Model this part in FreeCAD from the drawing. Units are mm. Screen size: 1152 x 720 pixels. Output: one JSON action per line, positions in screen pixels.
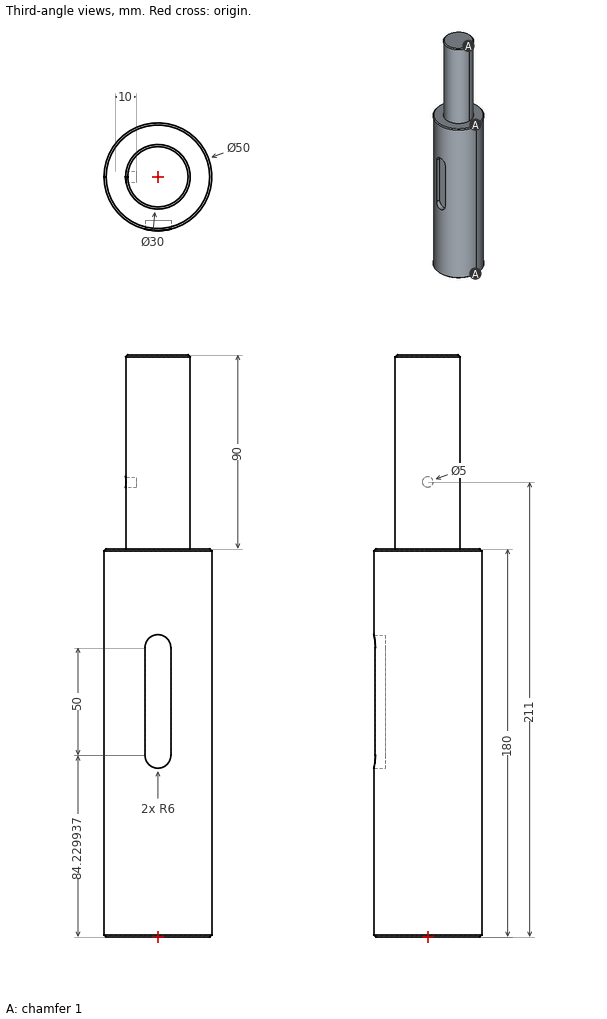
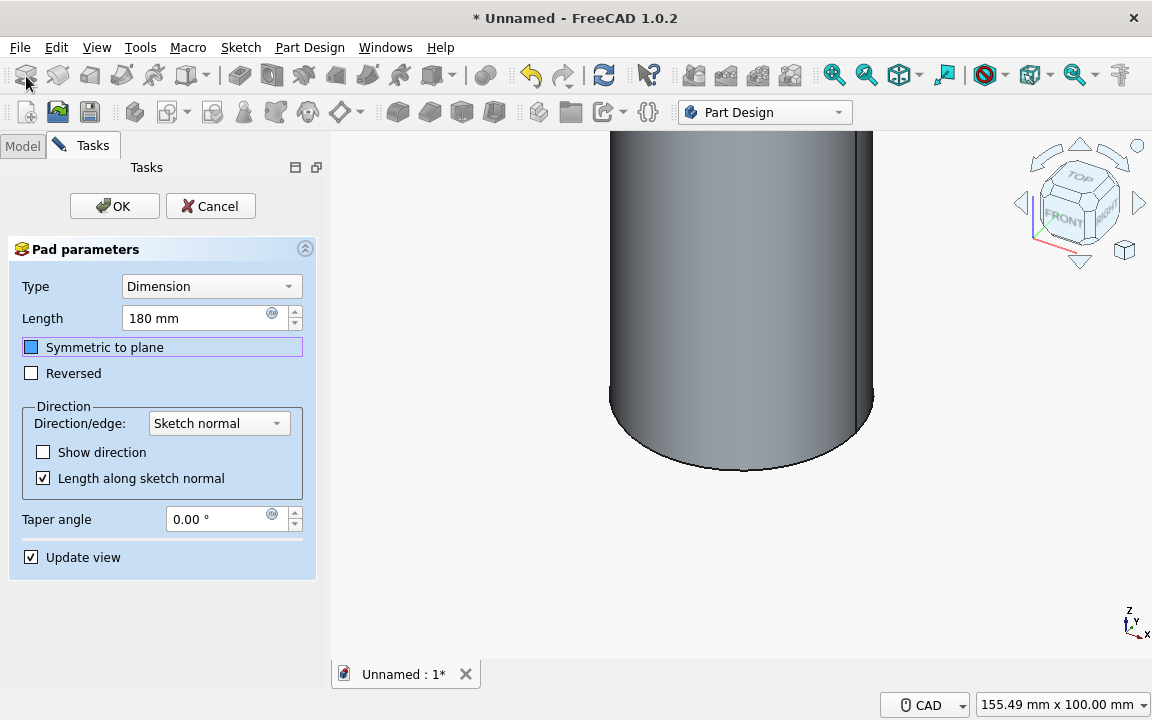
{"action": "left_click", "coordinate": [115, 206]}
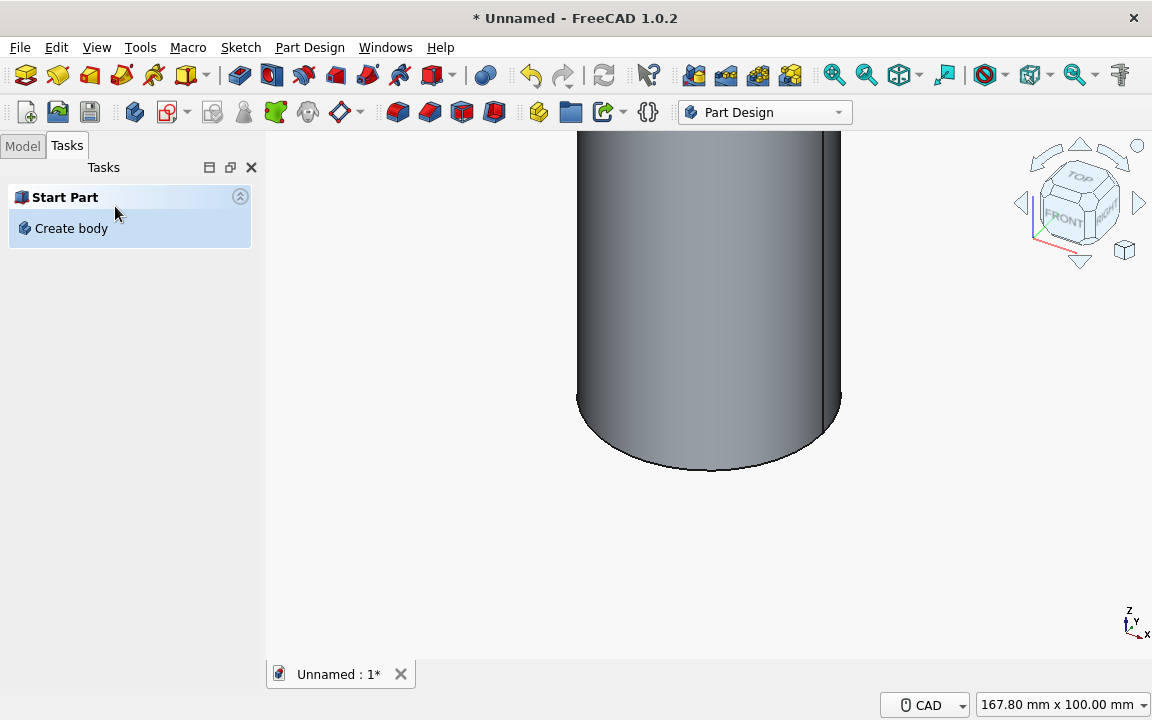
{"action": "key", "text": "v f"}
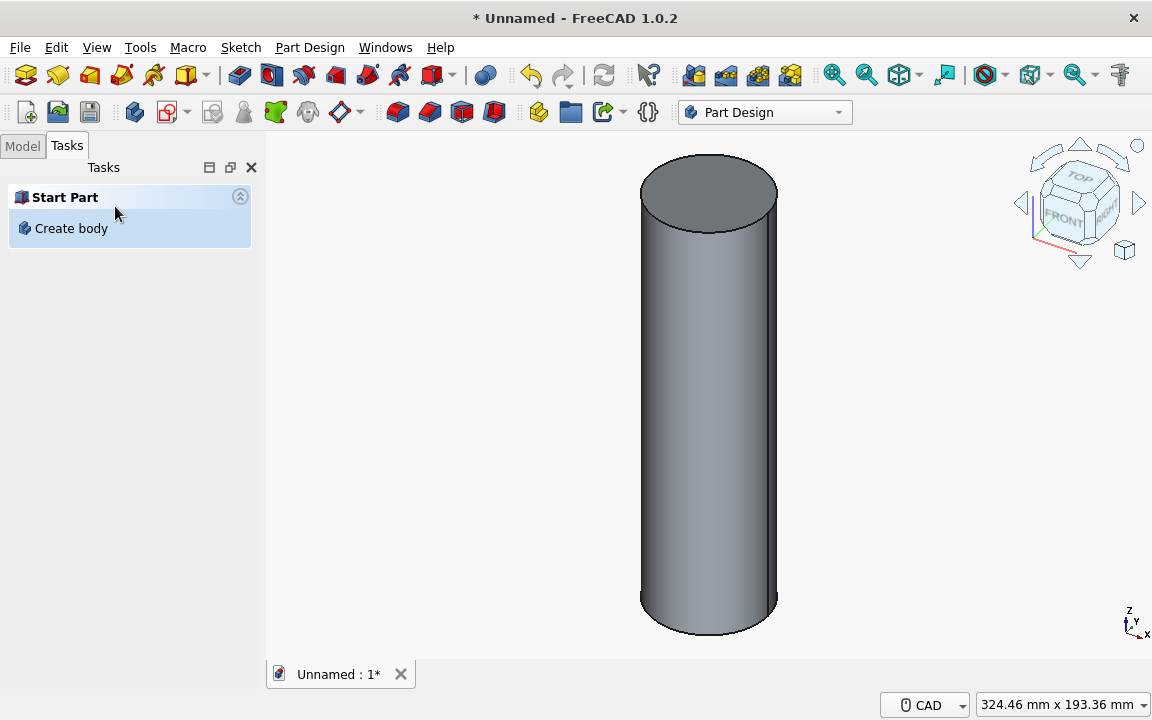
{"action": "left_click", "coordinate": [709, 193]}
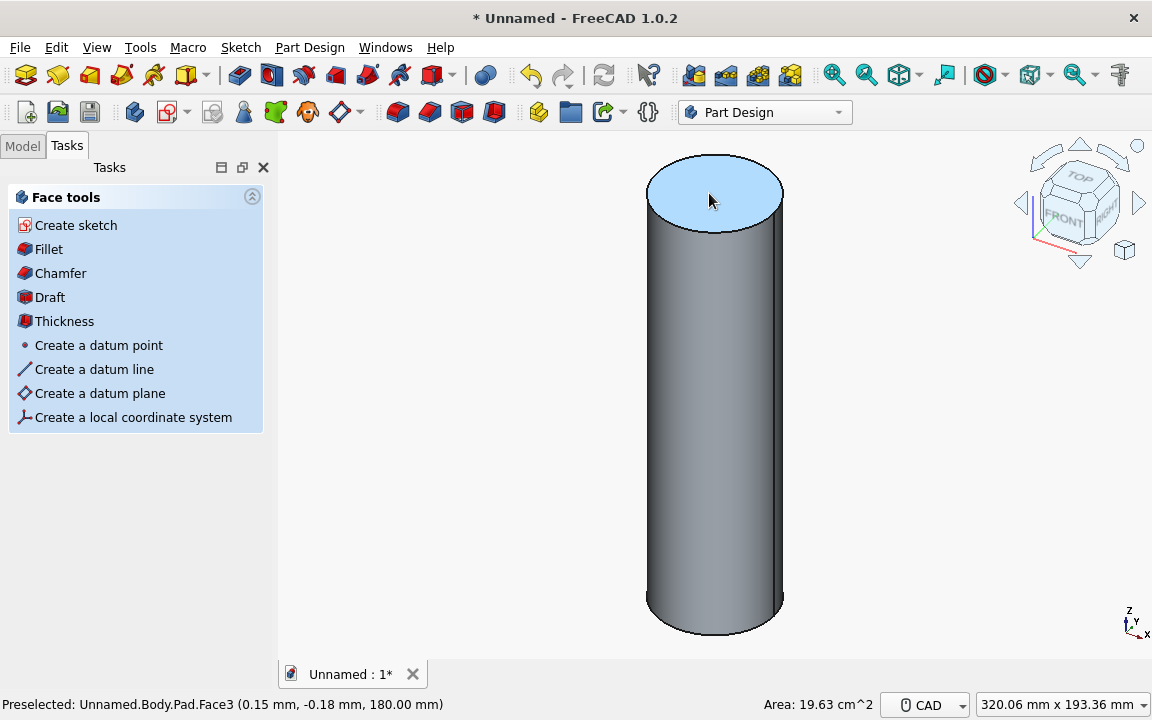
{"action": "left_click", "coordinate": [168, 112]}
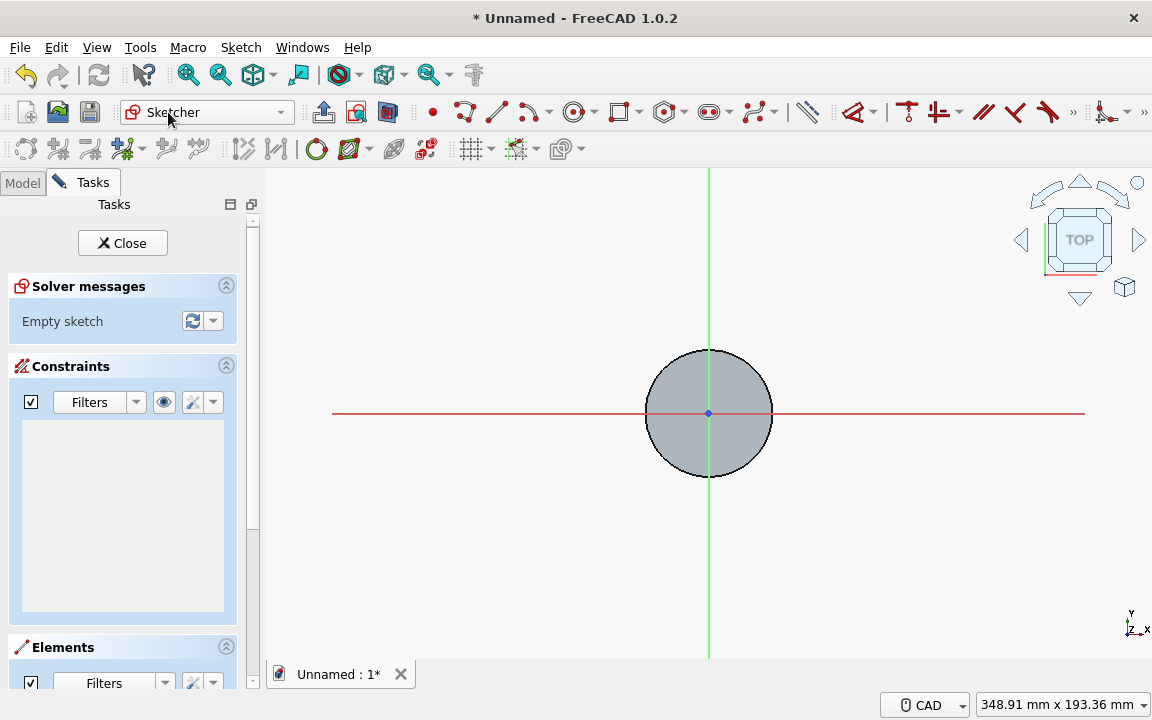
{"action": "scroll", "coordinate": [731, 414], "scroll_direction": "up", "scroll_amount": 7}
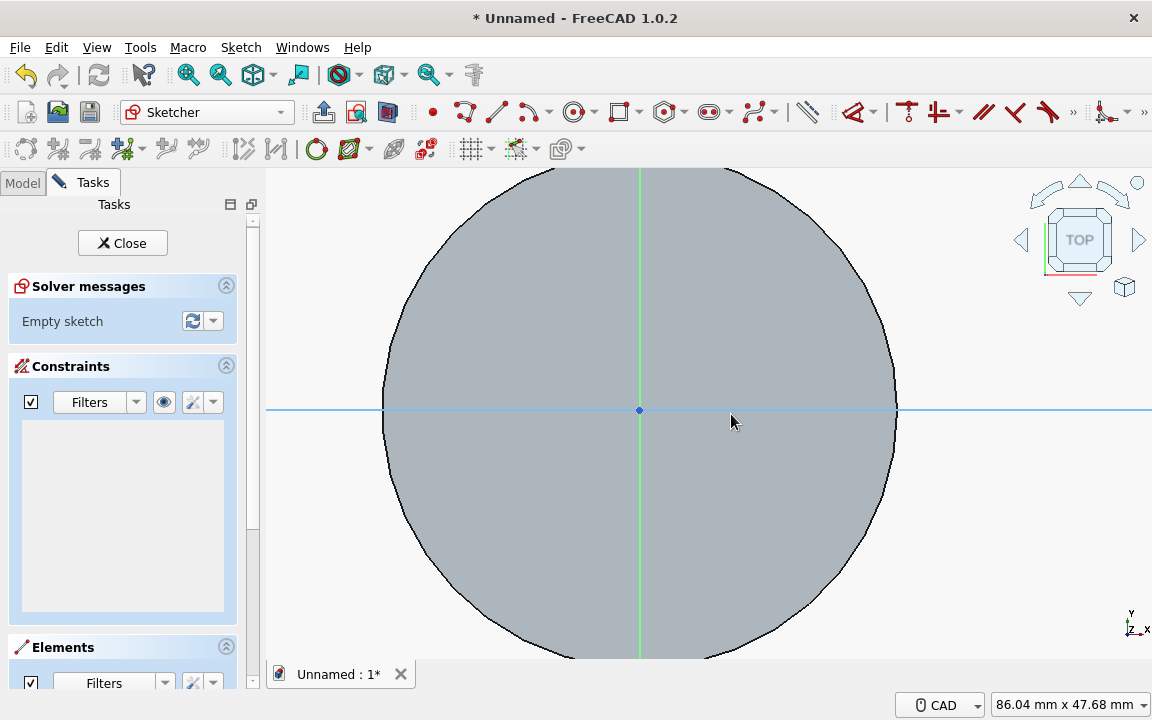
{"action": "key", "text": "g c"}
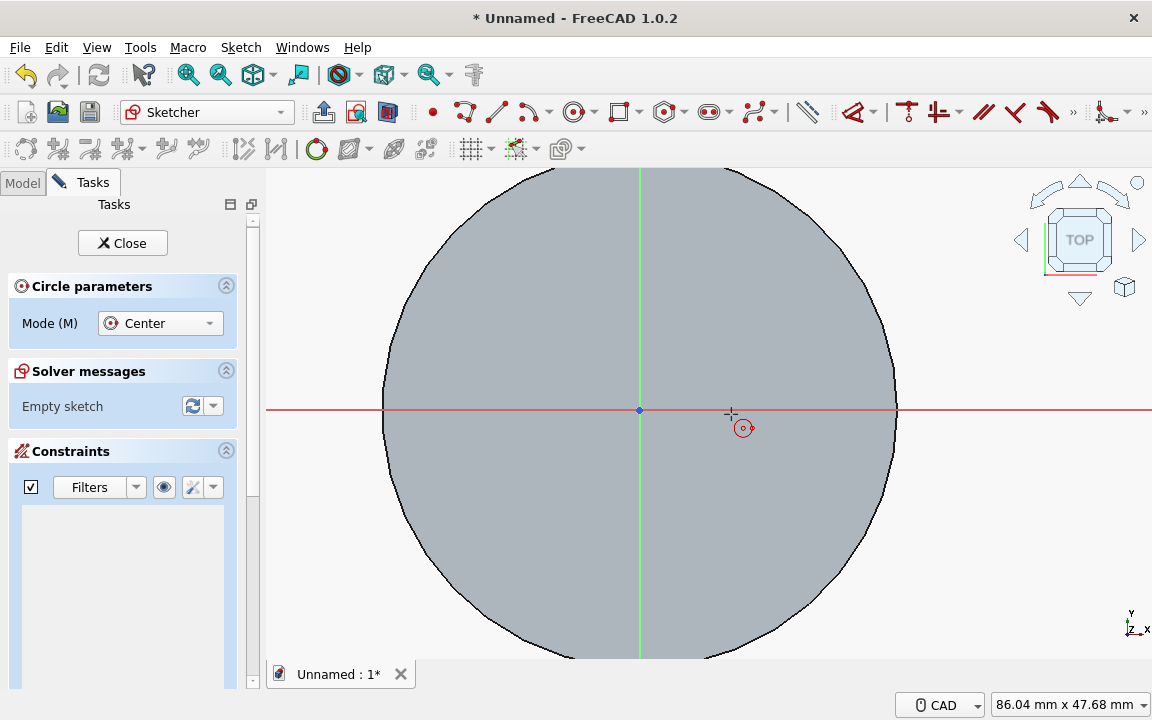
{"action": "left_click", "coordinate": [640, 410]}
{"action": "left_click", "coordinate": [749, 301]}
{"action": "key", "text": "Escape"}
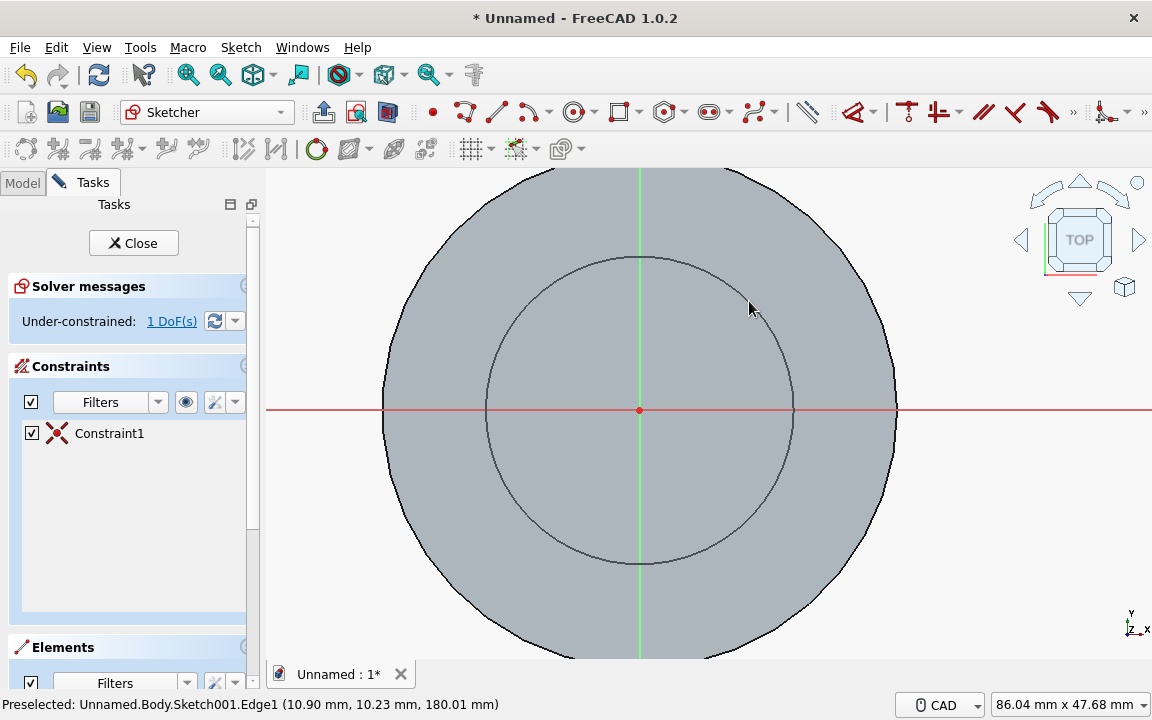
{"action": "key", "text": "d"}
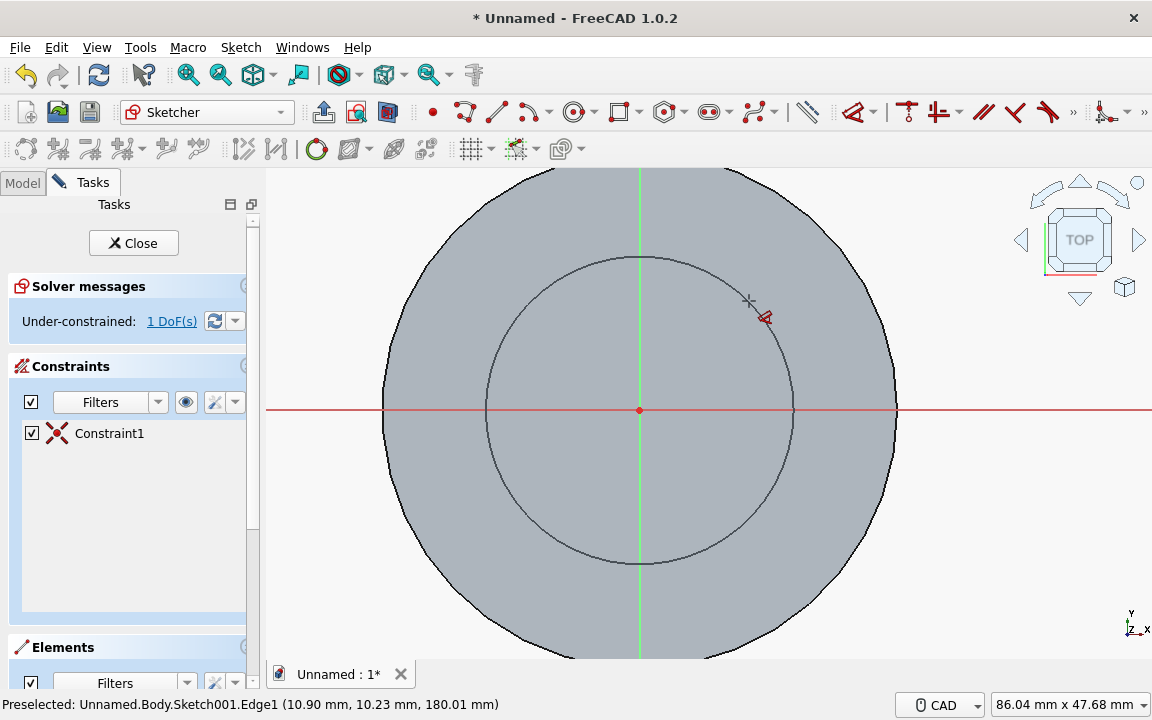
{"action": "left_click", "coordinate": [748, 301]}
{"action": "left_click", "coordinate": [771, 278]}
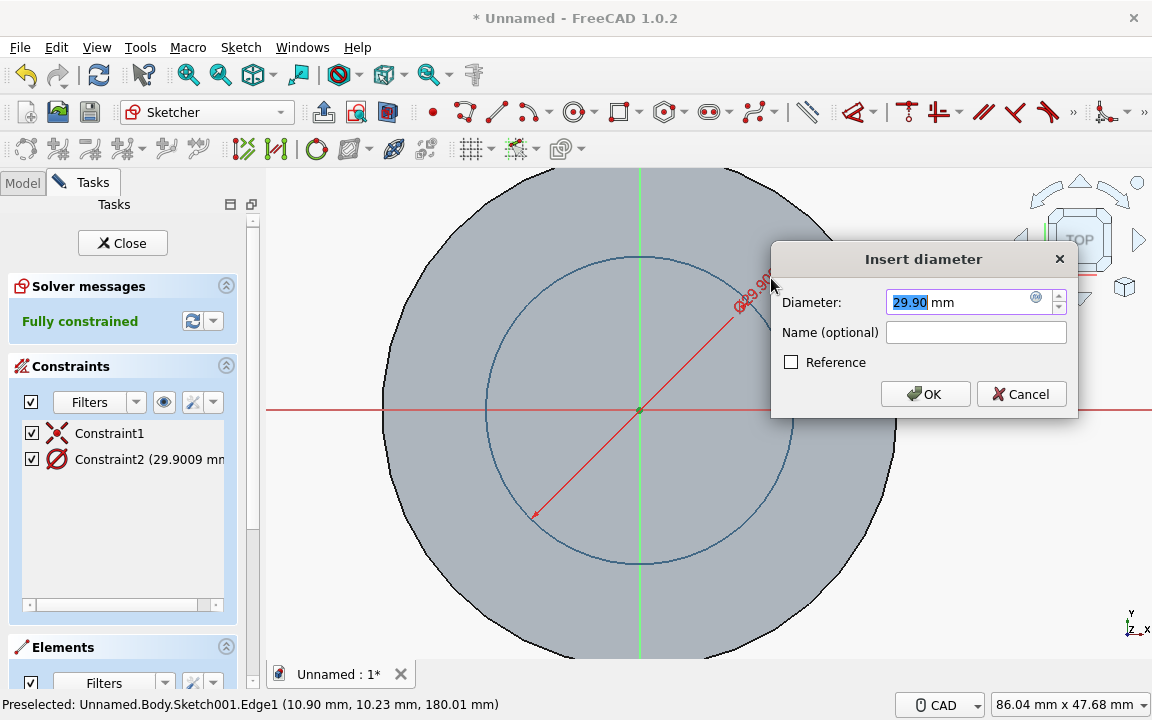
{"action": "type", "text": "30"}
{"action": "key", "text": "Return"}
{"action": "key", "text": "Escape"}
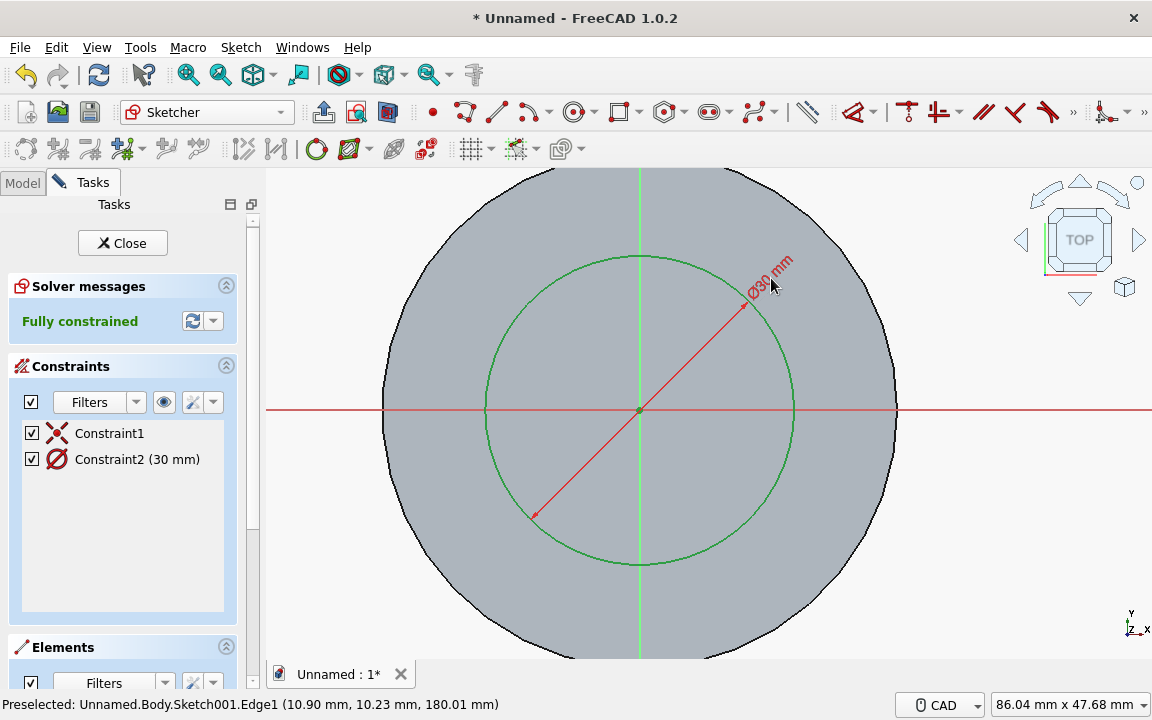
{"action": "left_click", "coordinate": [123, 243]}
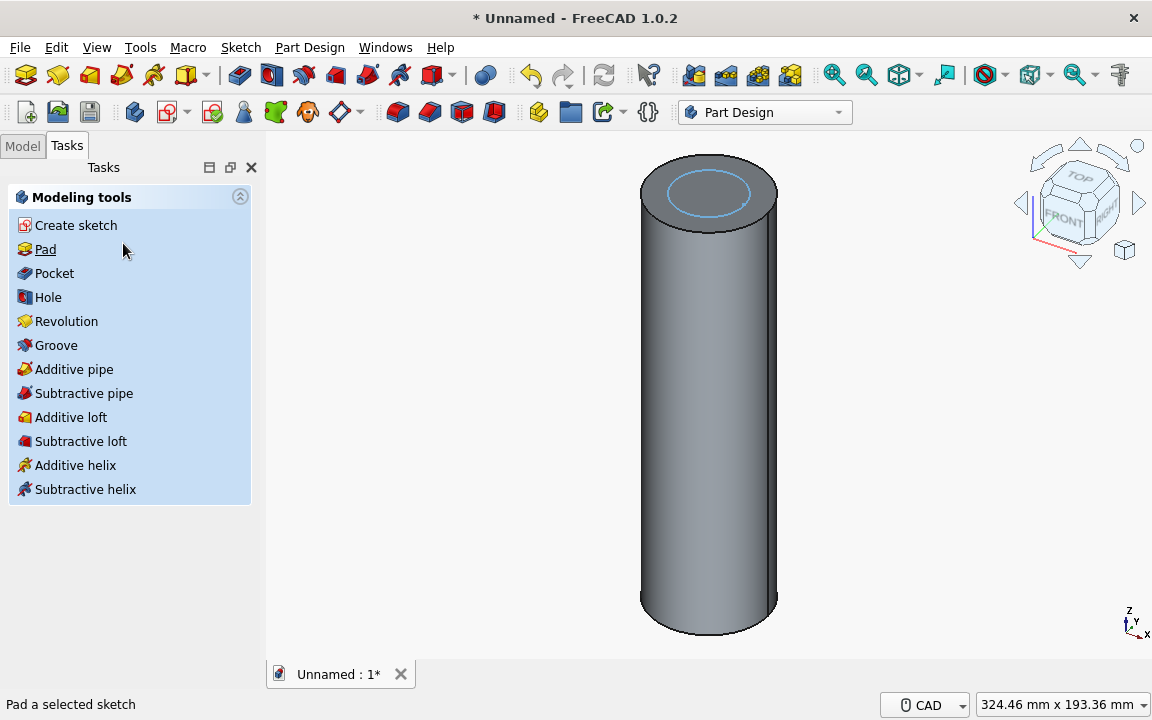
{"action": "left_click", "coordinate": [26, 76]}